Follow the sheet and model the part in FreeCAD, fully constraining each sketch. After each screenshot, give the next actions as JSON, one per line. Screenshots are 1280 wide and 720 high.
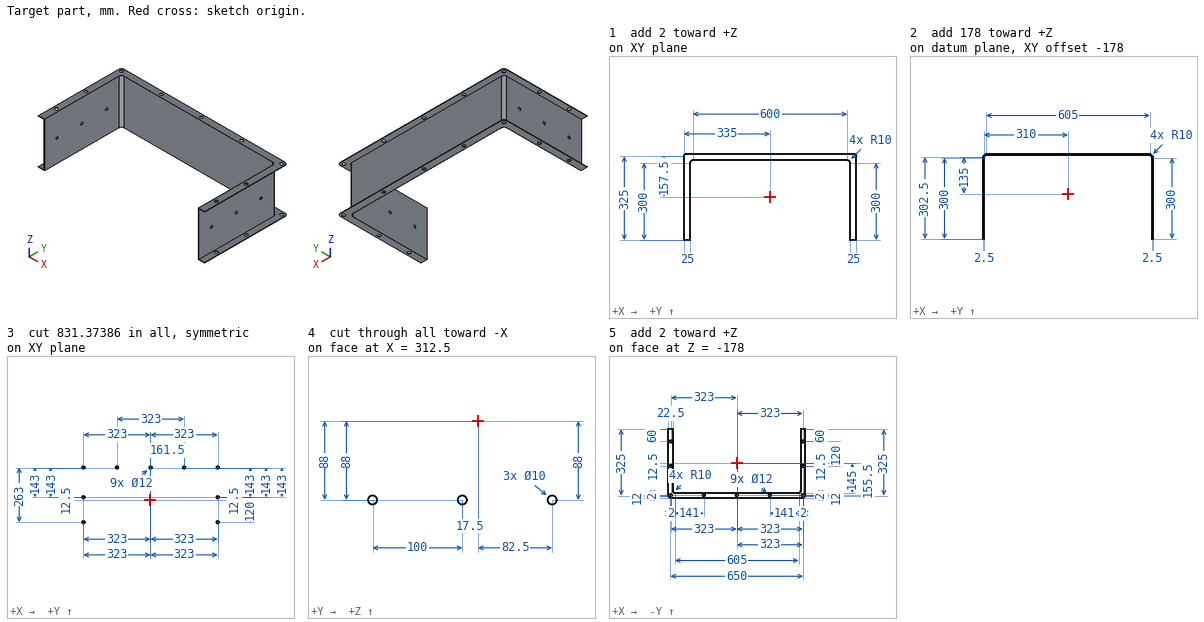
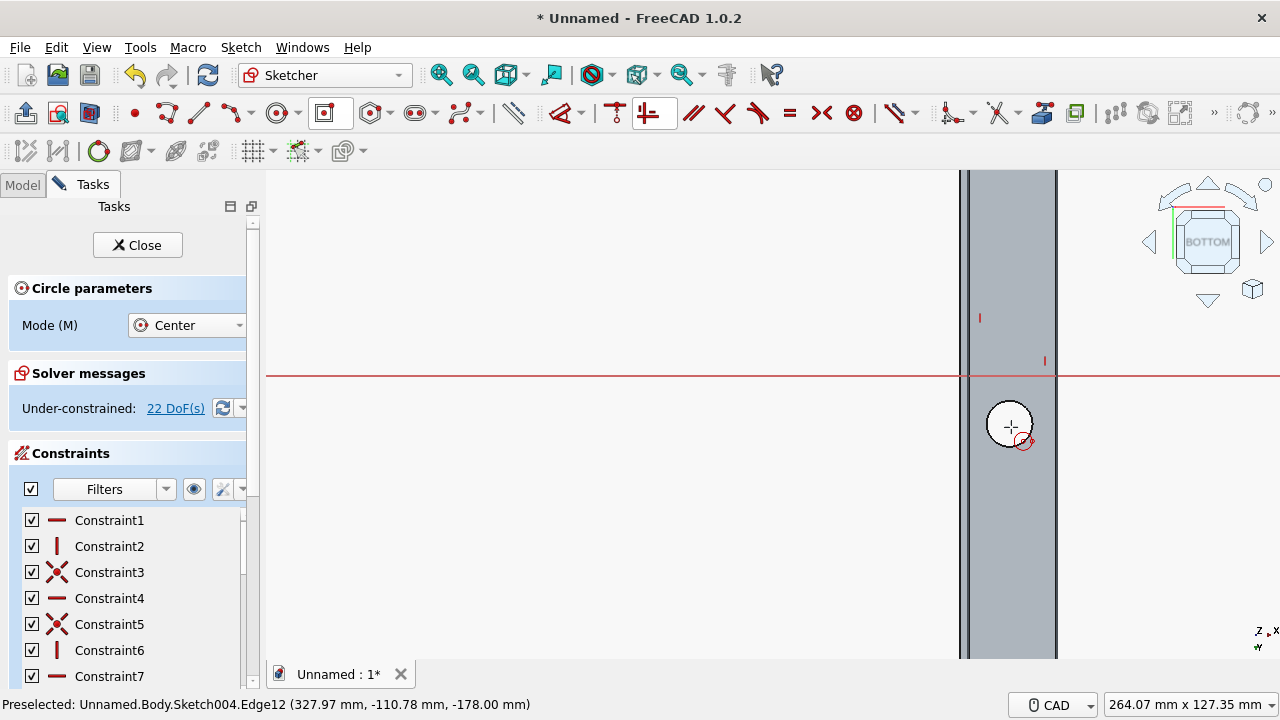
{"action": "left_click", "coordinate": [1010, 424]}
{"action": "mouse_move", "coordinate": [1026, 408]}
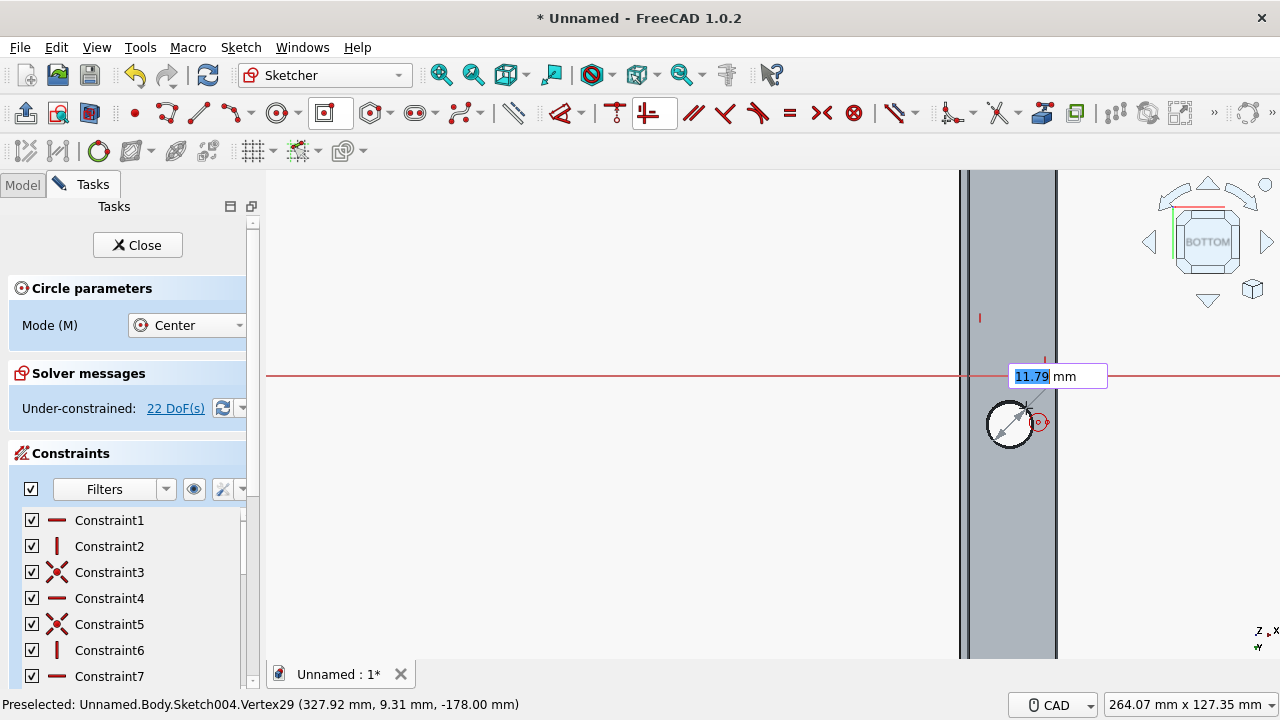
{"action": "type", "text": "12"}
{"action": "key", "text": "Return"}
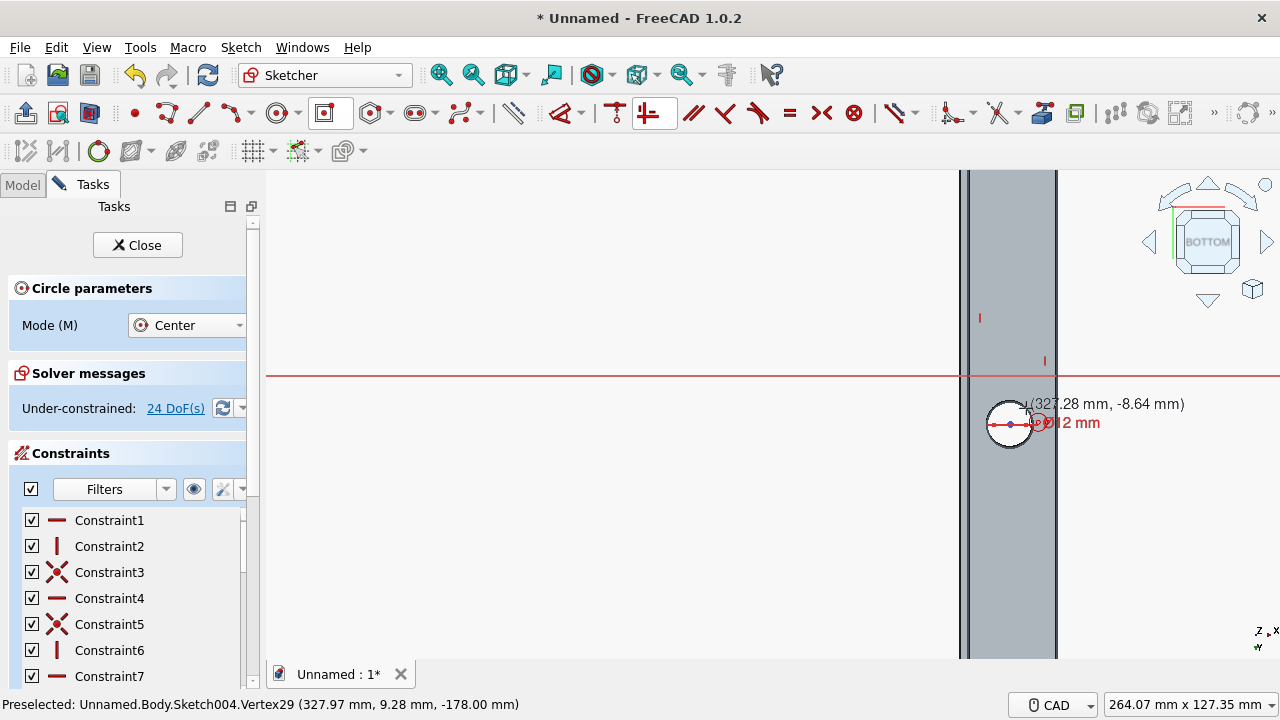
{"action": "scroll", "coordinate": [1011, 427], "scroll_direction": "down", "scroll_amount": 7}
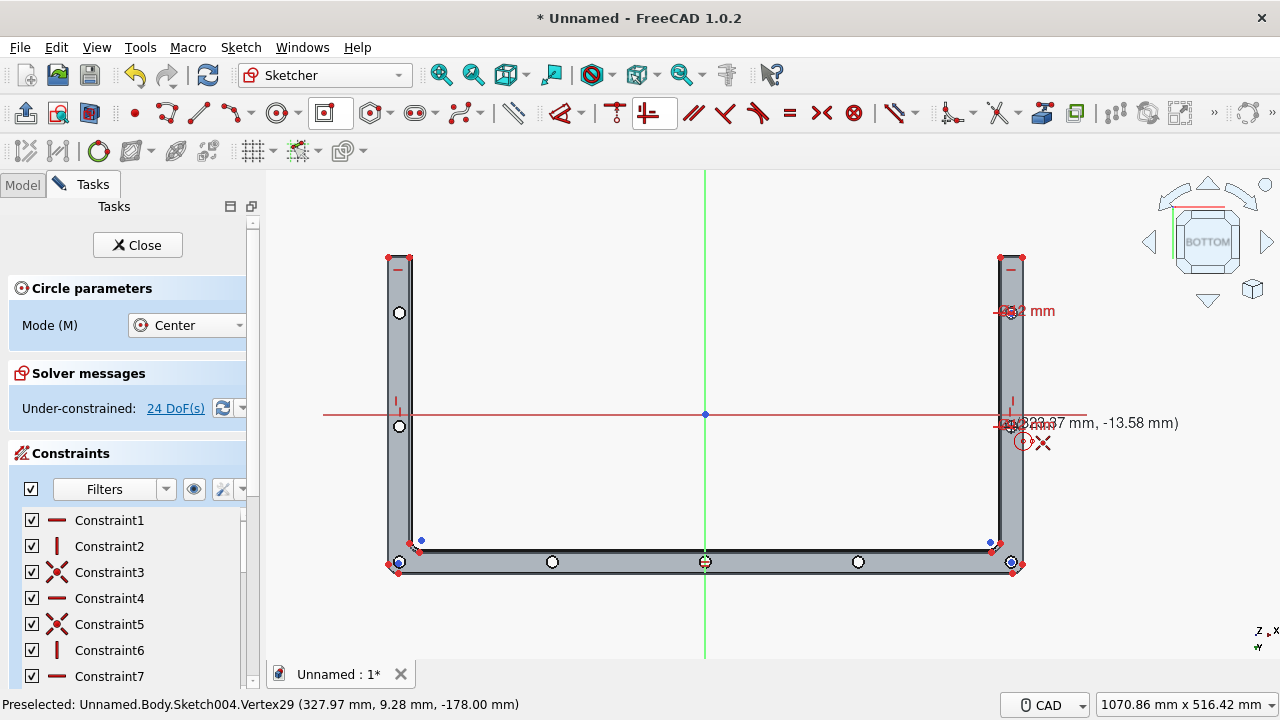
{"action": "scroll", "coordinate": [399, 313], "scroll_direction": "up", "scroll_amount": 7}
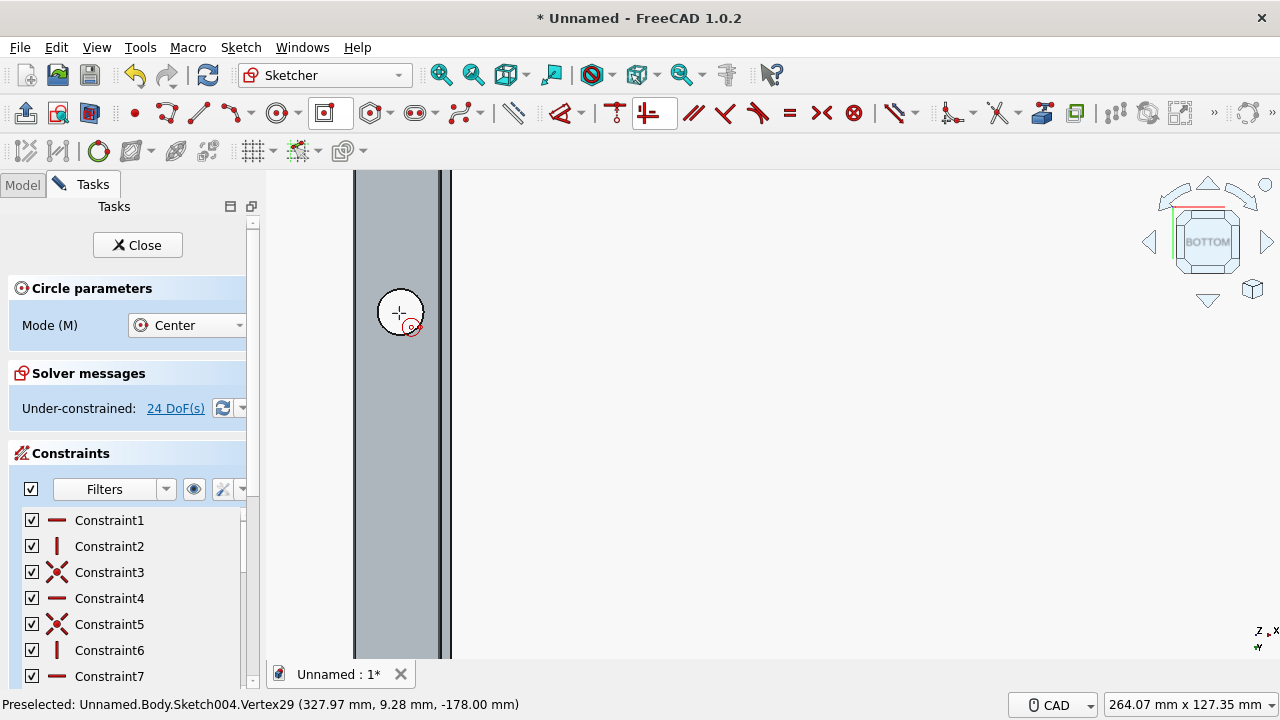
{"action": "left_click", "coordinate": [401, 312]}
{"action": "mouse_move", "coordinate": [417, 296]}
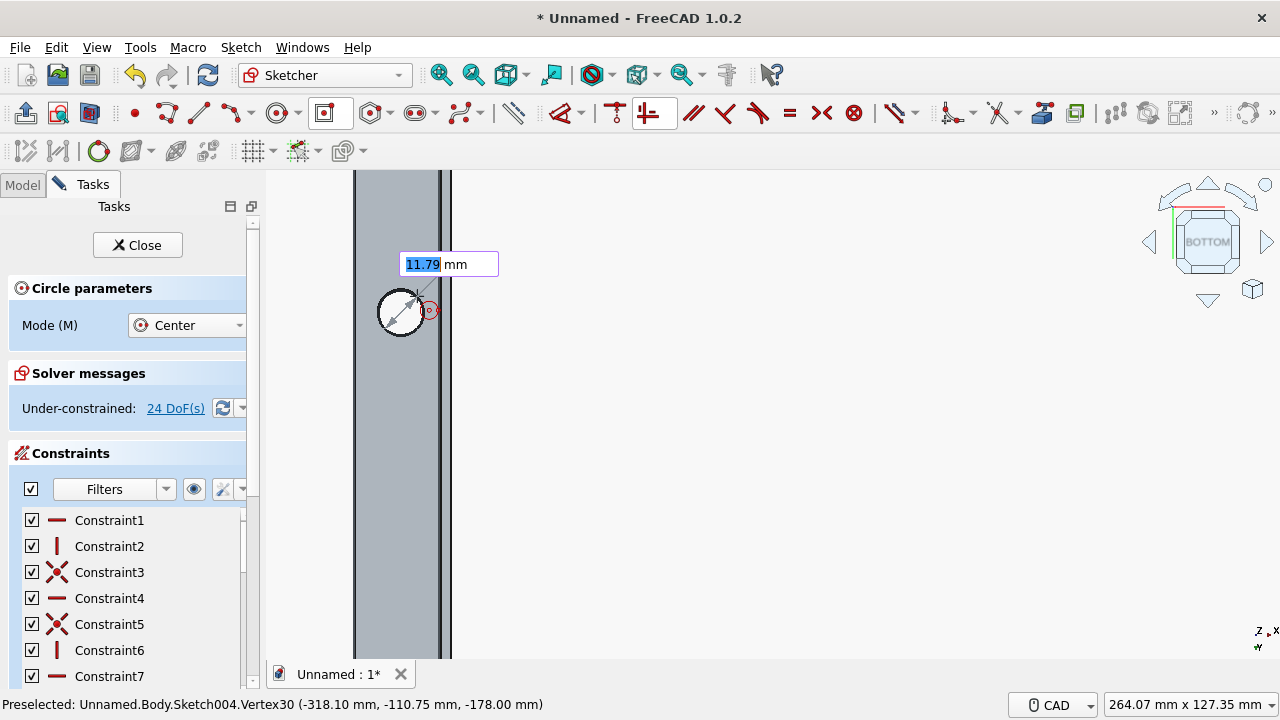
{"action": "type", "text": "12"}
{"action": "key", "text": "Return"}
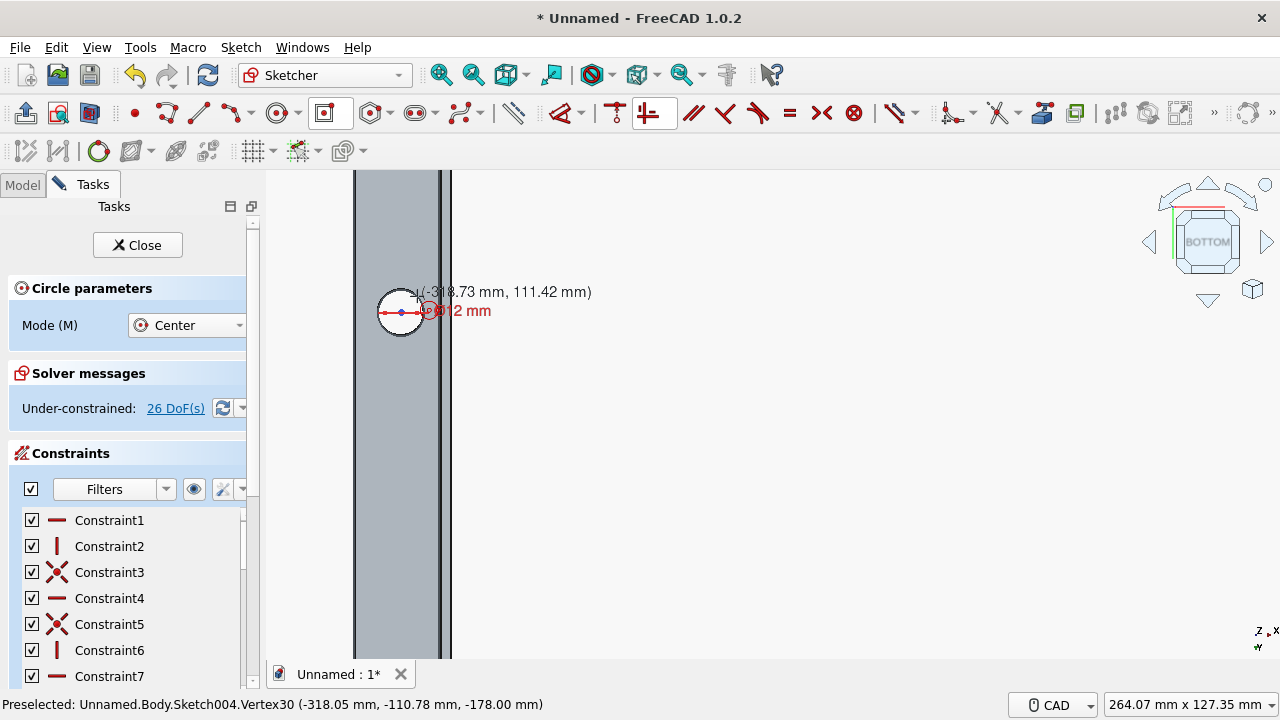
{"action": "scroll", "coordinate": [398, 313], "scroll_direction": "down", "scroll_amount": 7}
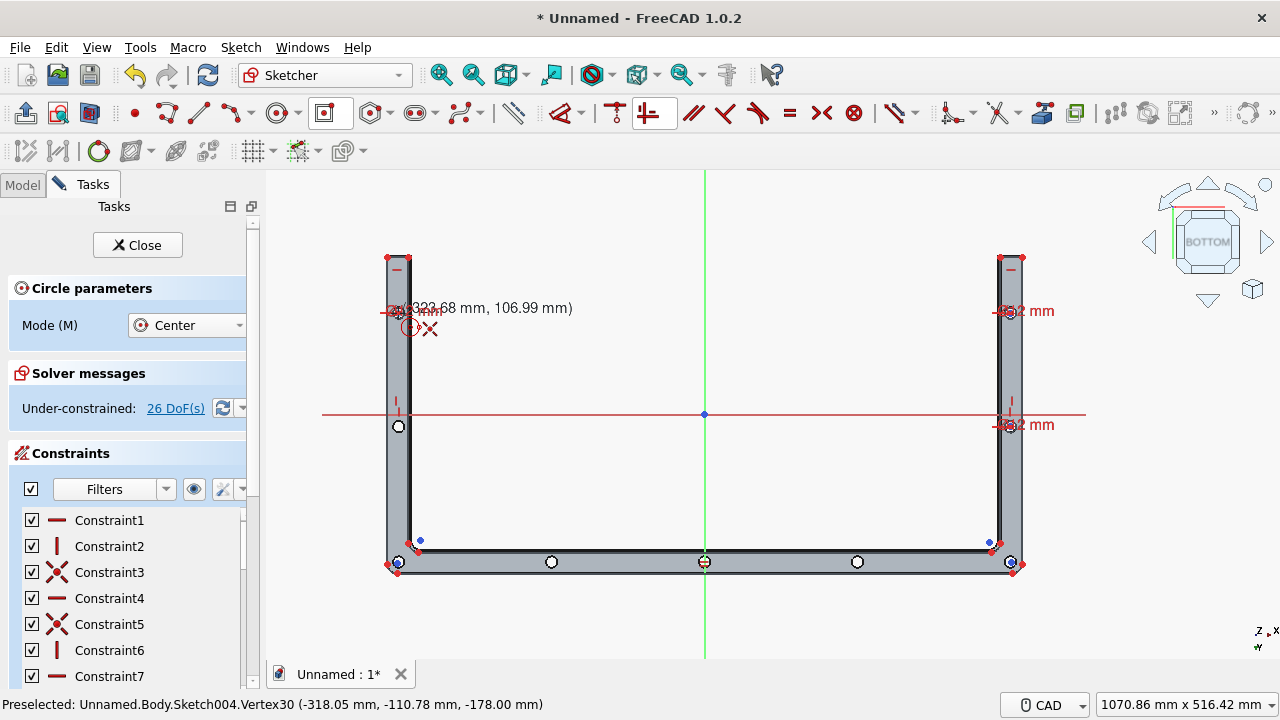
{"action": "scroll", "coordinate": [399, 427], "scroll_direction": "up", "scroll_amount": 7}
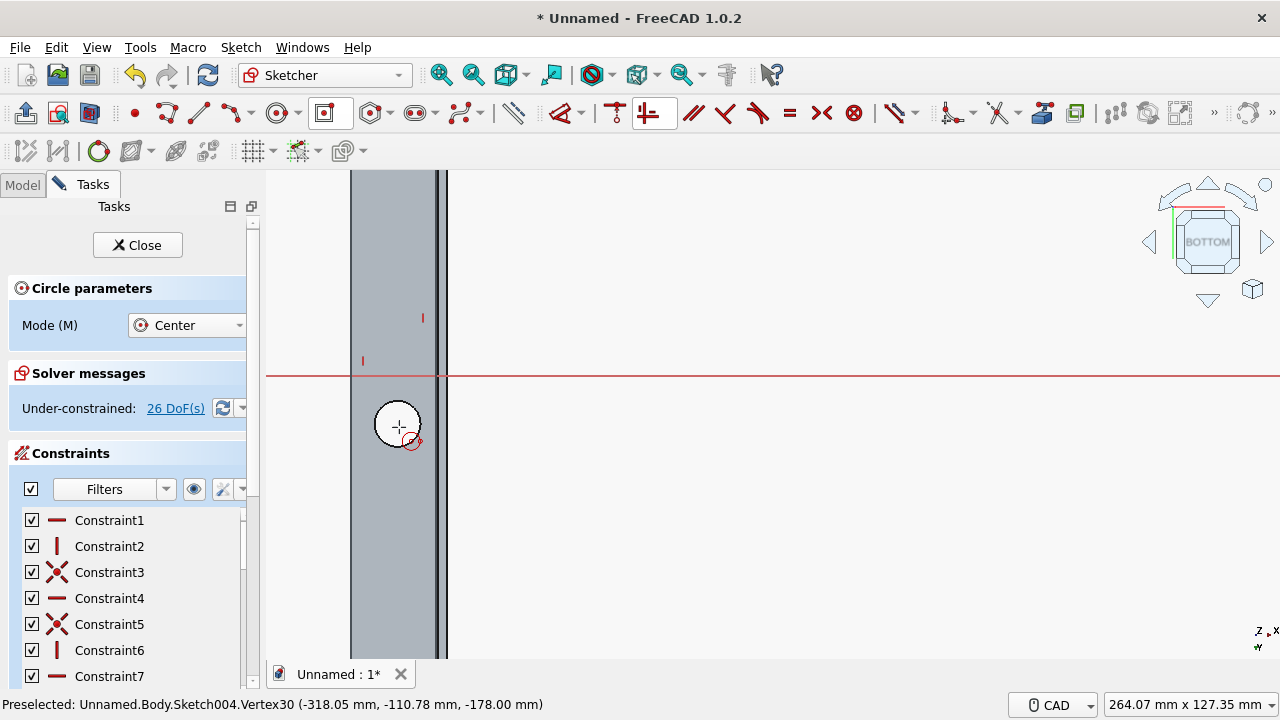
{"action": "left_click", "coordinate": [398, 424]}
{"action": "mouse_move", "coordinate": [414, 408]}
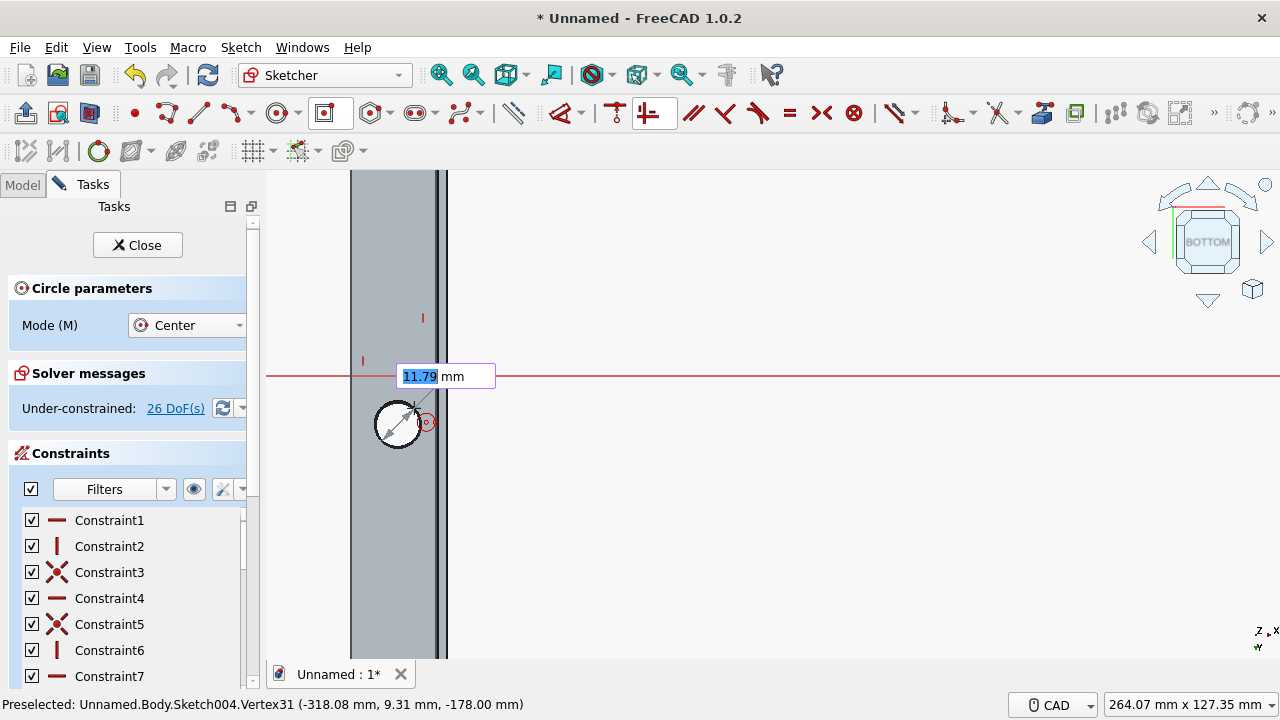
{"action": "type", "text": "12"}
{"action": "key", "text": "Return"}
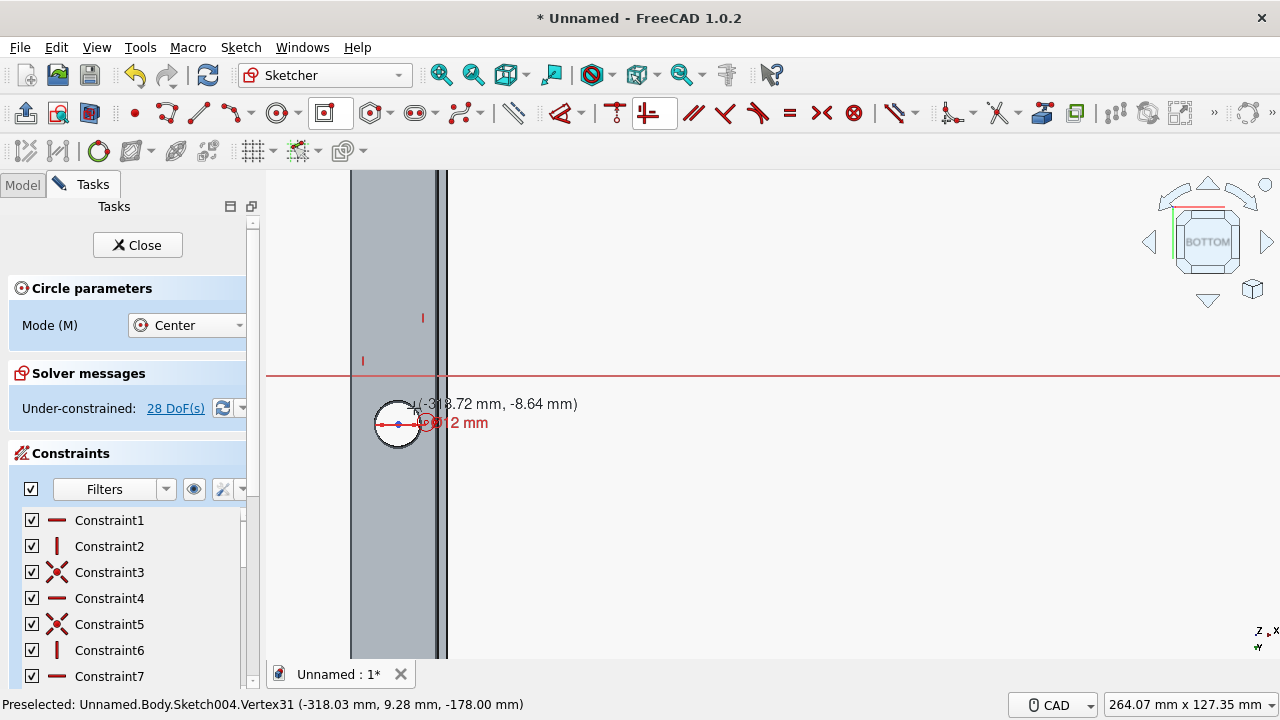
{"action": "scroll", "coordinate": [399, 427], "scroll_direction": "down", "scroll_amount": 7}